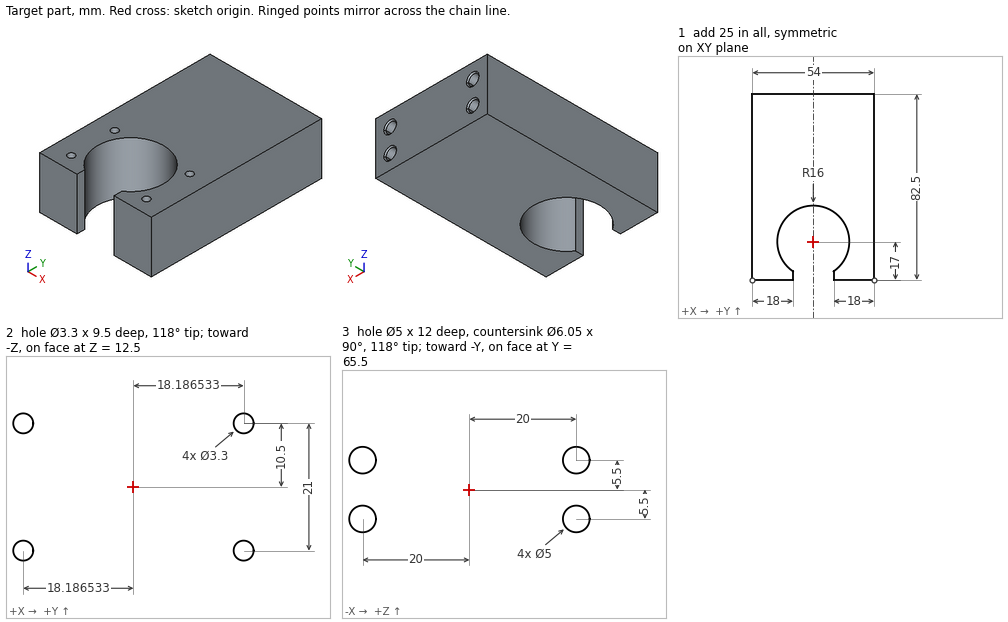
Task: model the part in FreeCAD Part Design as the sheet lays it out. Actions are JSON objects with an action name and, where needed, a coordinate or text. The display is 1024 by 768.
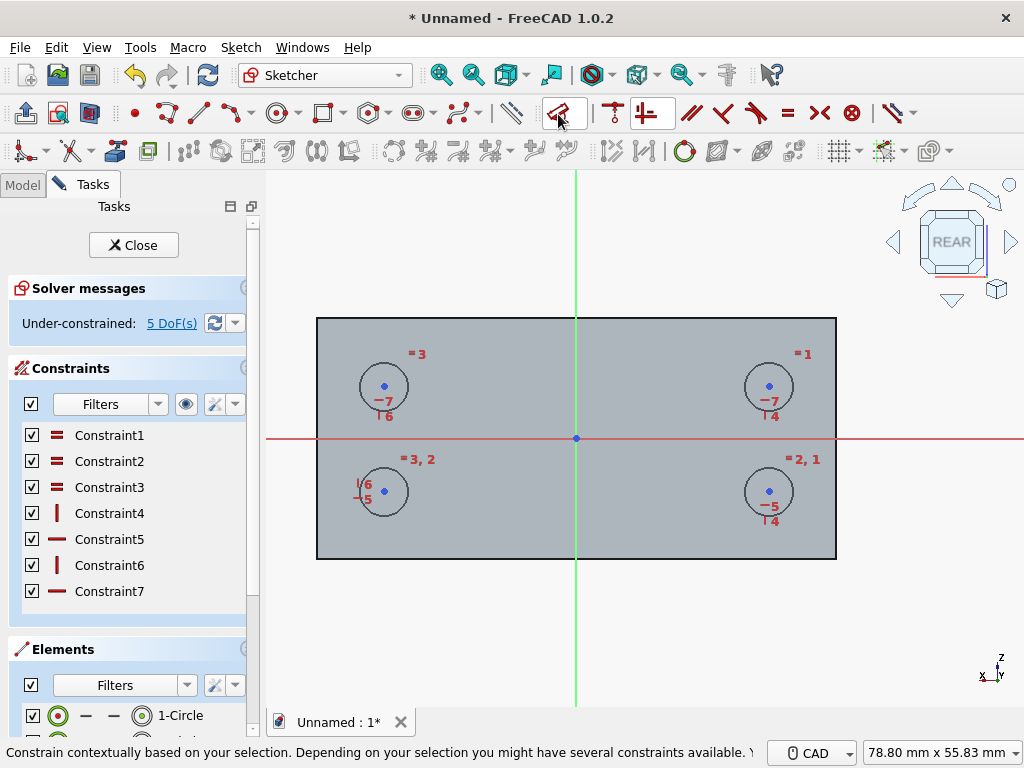
{"action": "left_click", "coordinate": [786, 370]}
{"action": "left_click", "coordinate": [809, 347]}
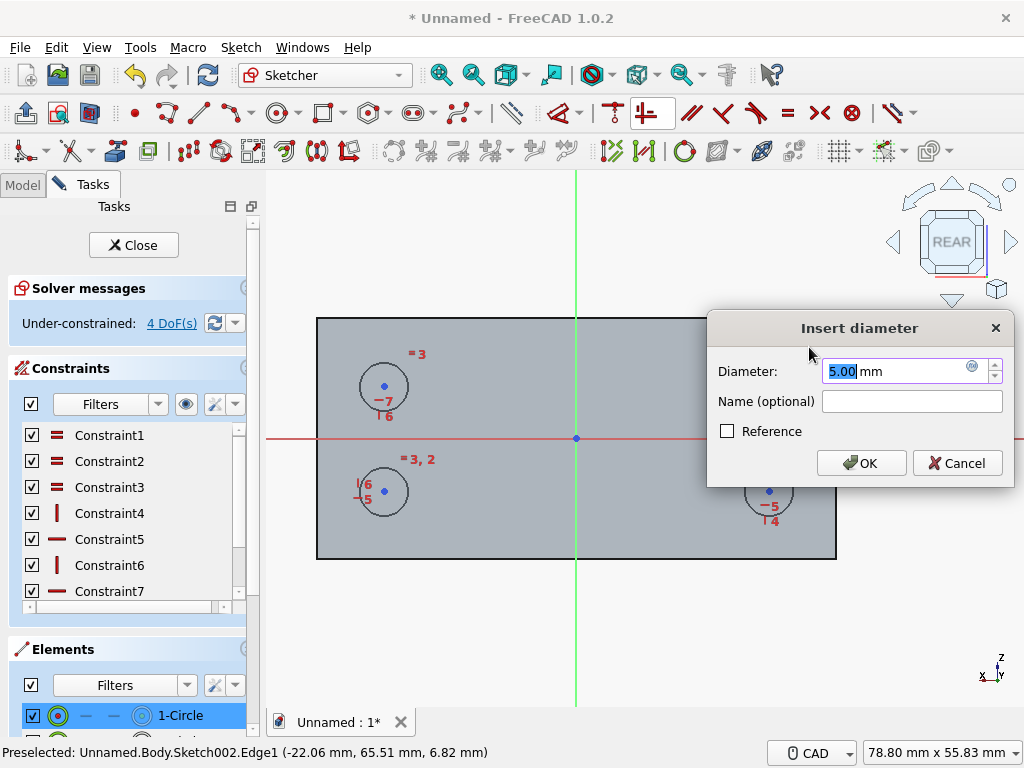
{"action": "type", "text": "5"}
{"action": "key", "text": "Return"}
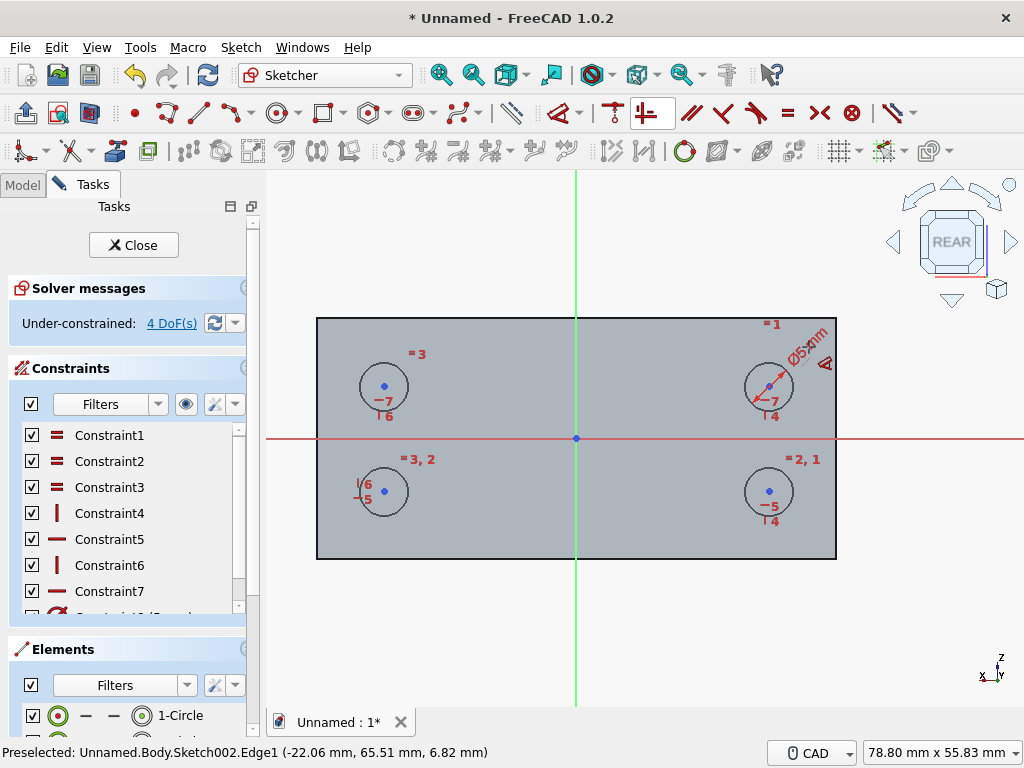
{"action": "left_click", "coordinate": [769, 387]}
{"action": "left_click", "coordinate": [673, 353]}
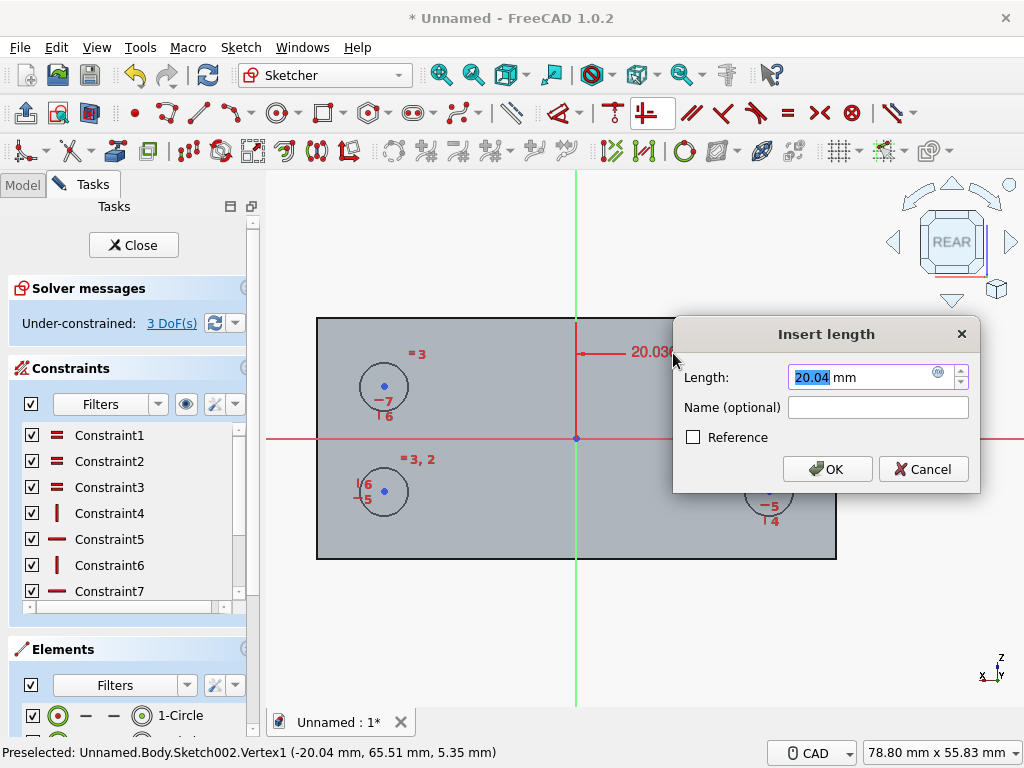
{"action": "type", "text": "20"}
{"action": "key", "text": "Return"}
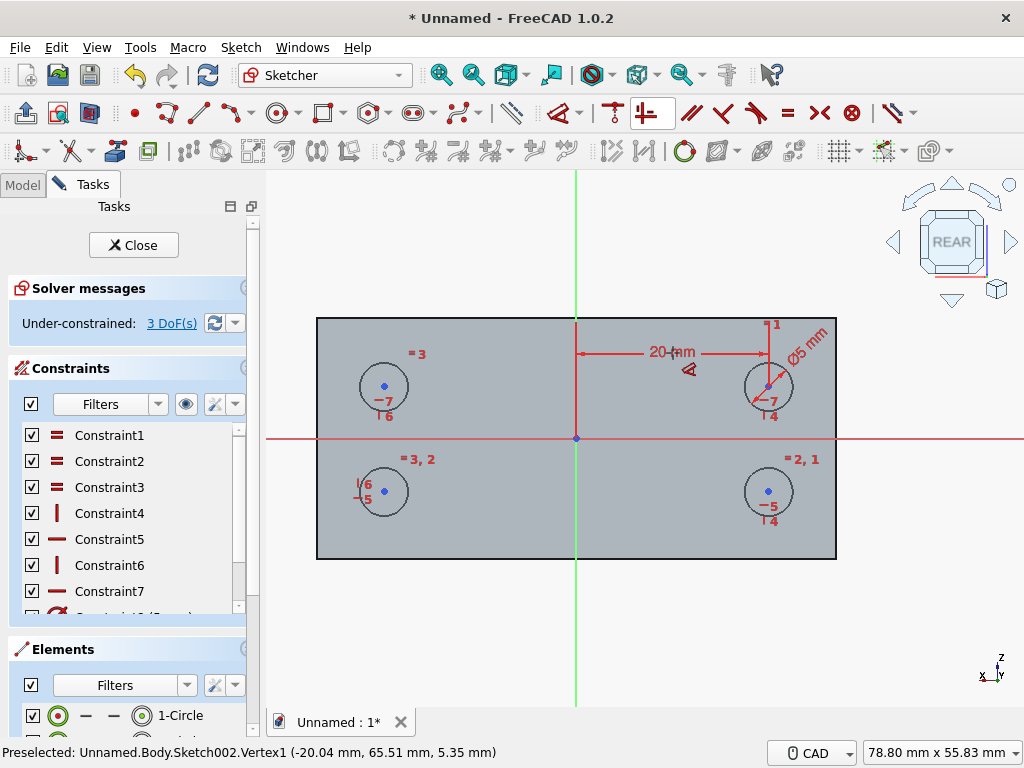
{"action": "left_click", "coordinate": [384, 492]}
{"action": "left_click", "coordinate": [480, 526]}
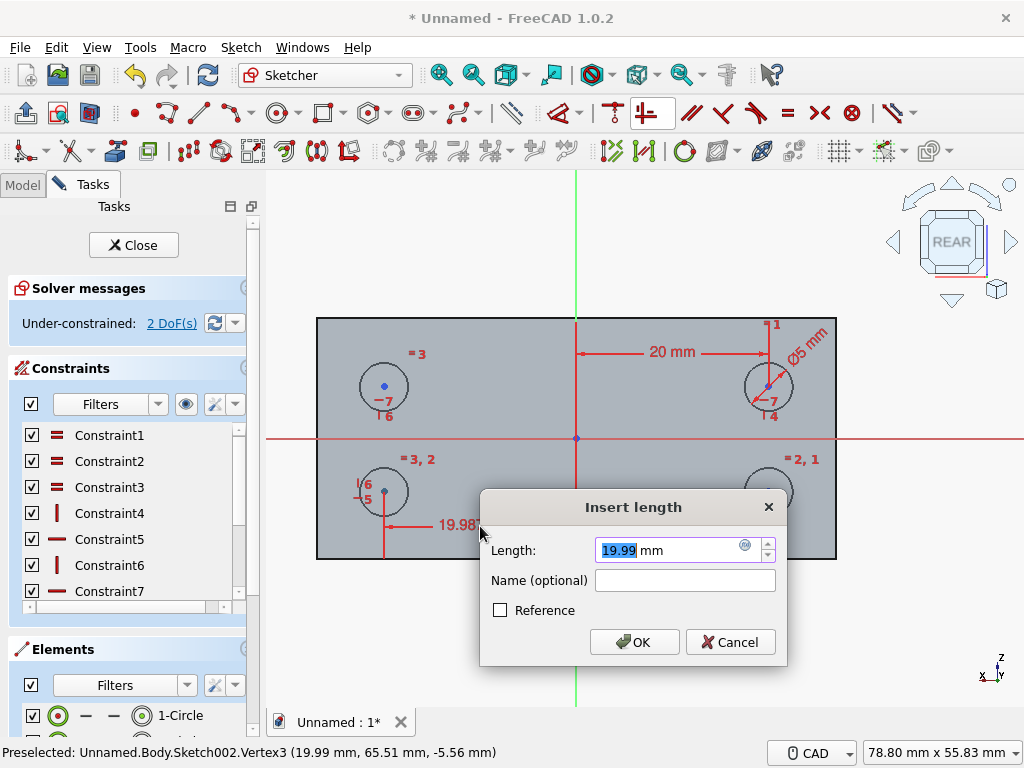
{"action": "type", "text": "20"}
{"action": "key", "text": "Return"}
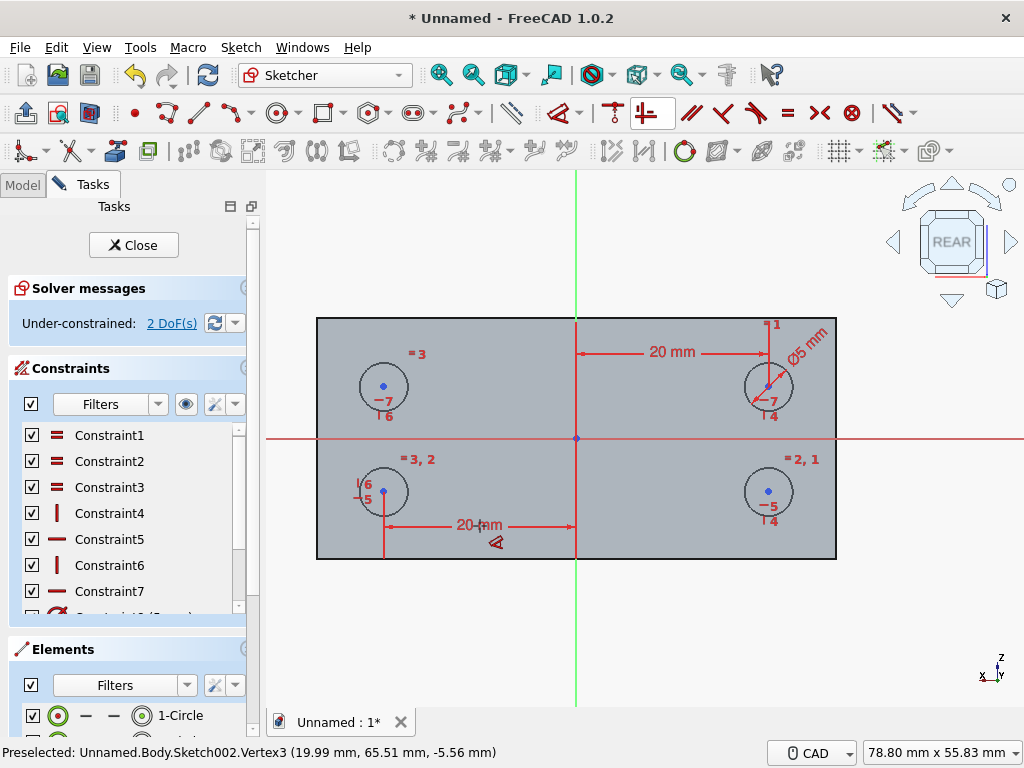
{"action": "left_click", "coordinate": [769, 387]}
{"action": "left_click", "coordinate": [803, 413]}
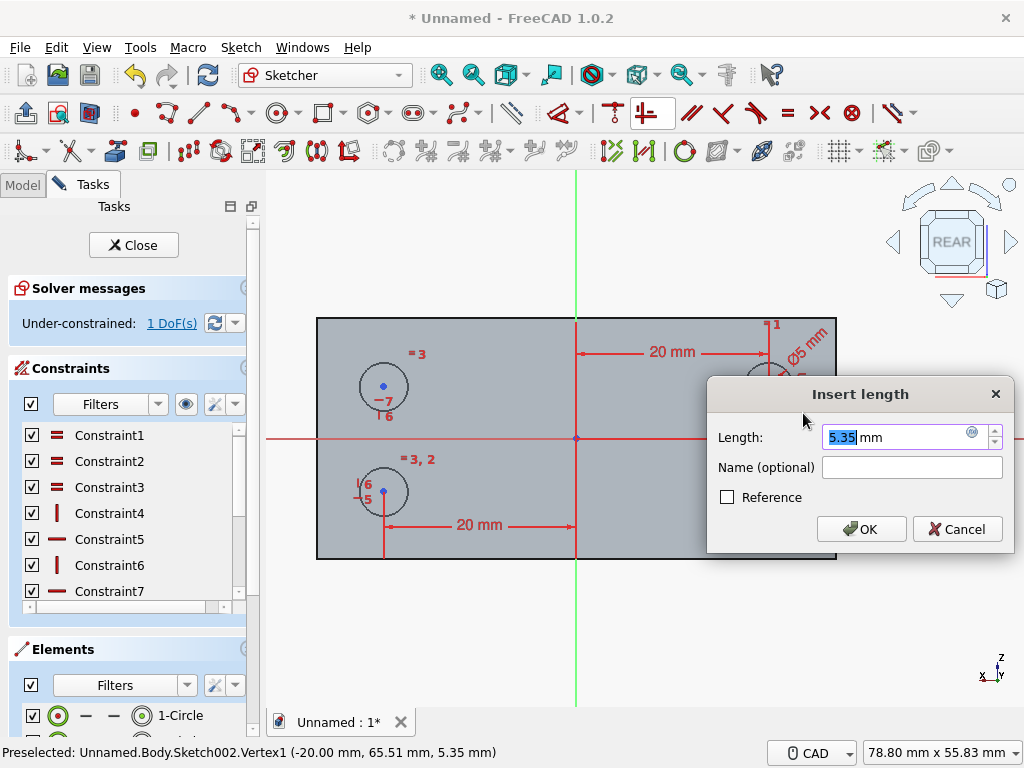
{"action": "type", "text": "5.5"}
{"action": "key", "text": "Return"}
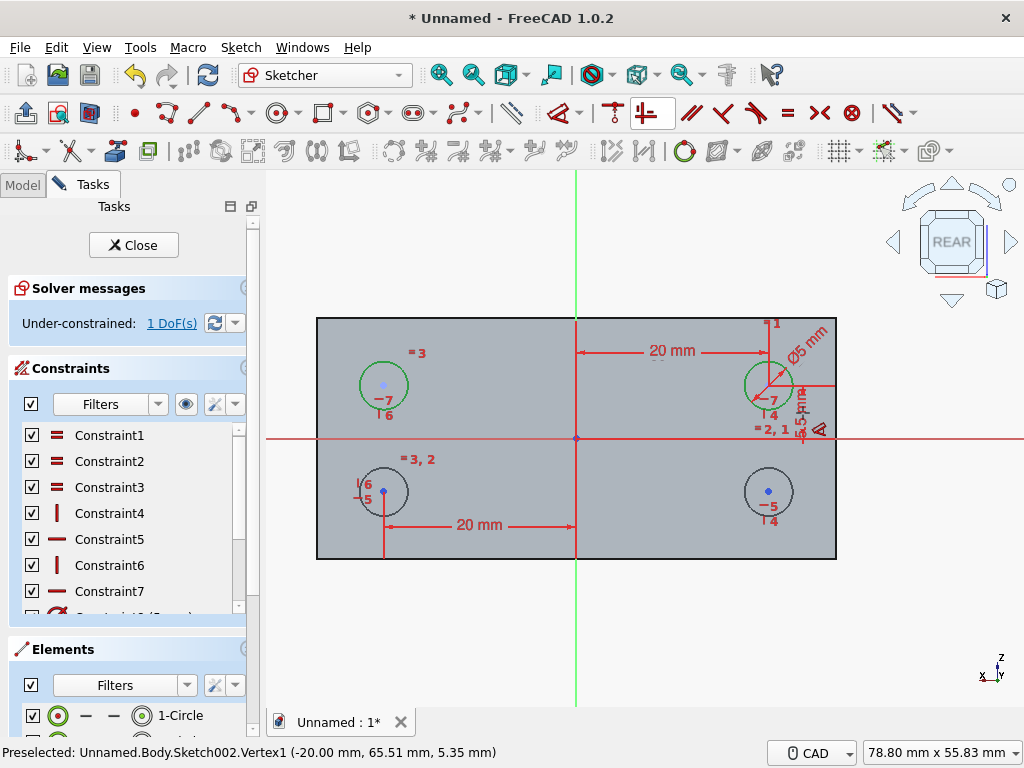
{"action": "left_click", "coordinate": [769, 492]}
{"action": "left_click", "coordinate": [803, 465]}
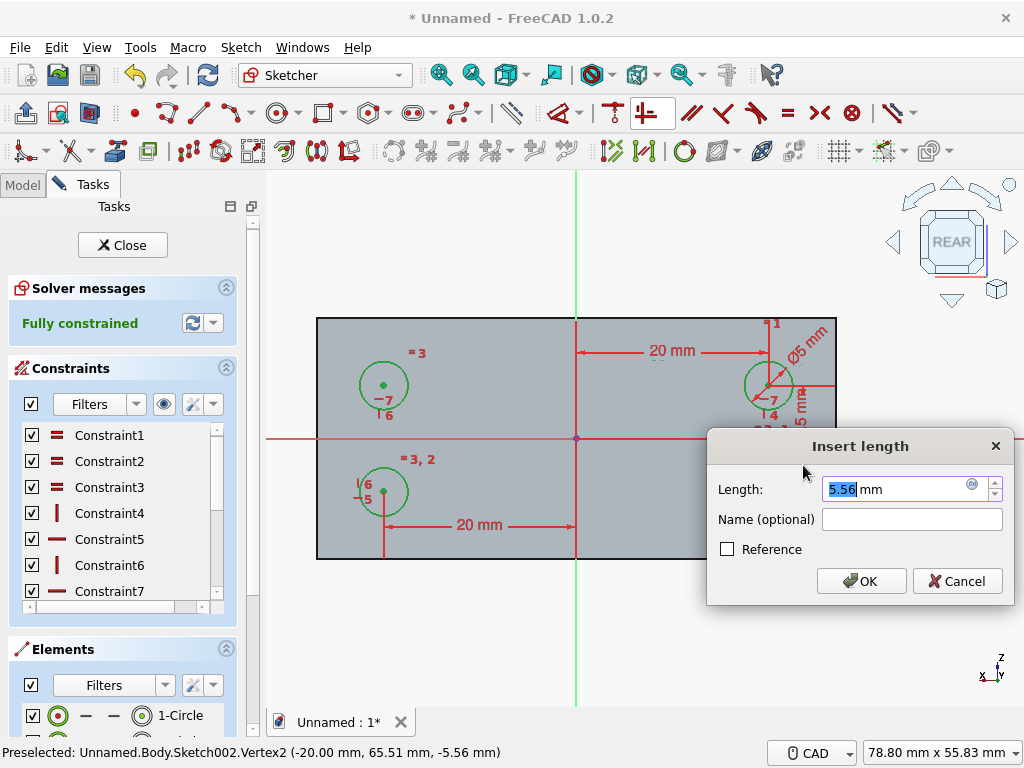
{"action": "type", "text": "5.5"}
{"action": "key", "text": "Return"}
{"action": "key", "text": "Escape"}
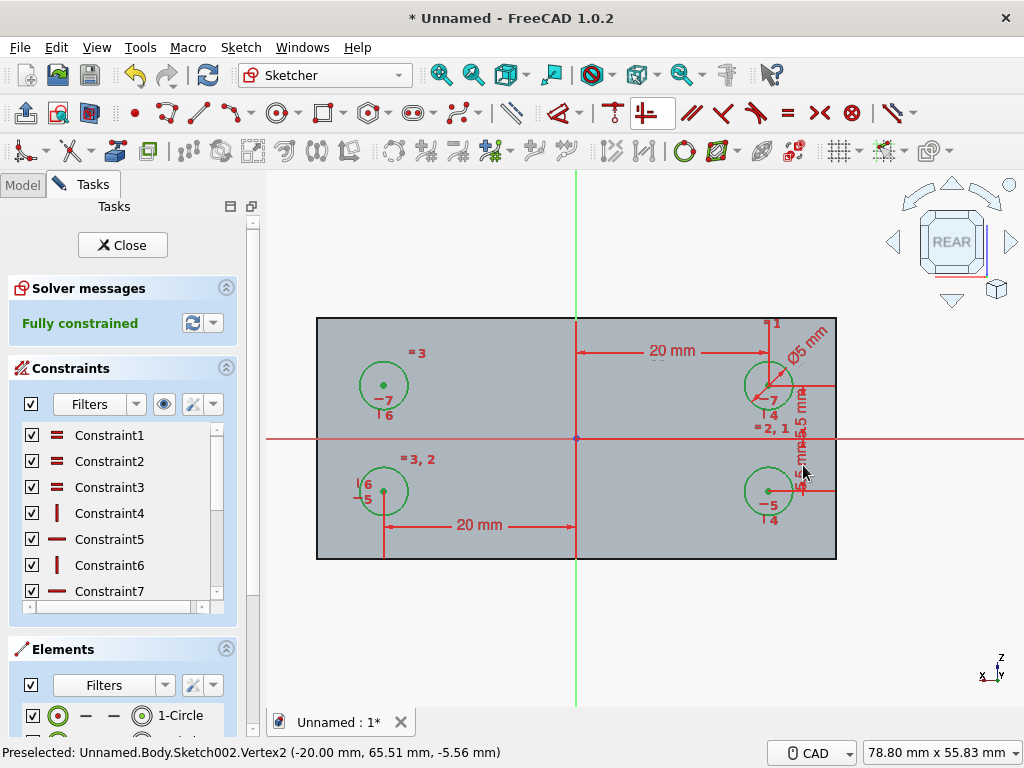
{"action": "left_click", "coordinate": [123, 245]}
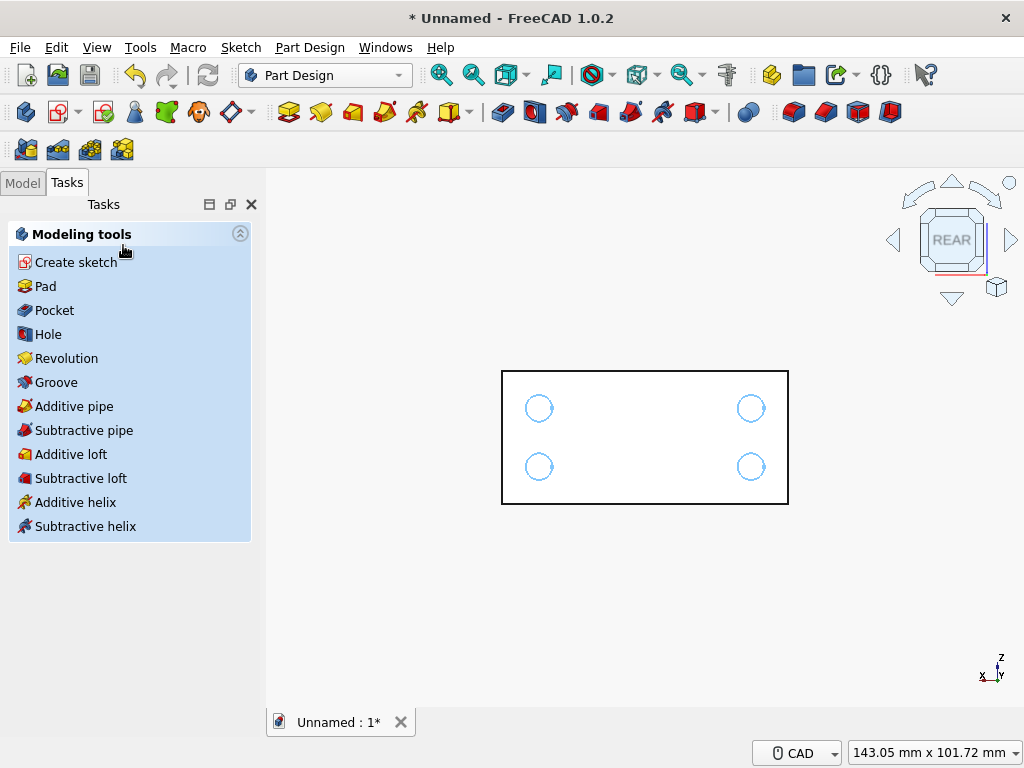
{"action": "left_click", "coordinate": [536, 112]}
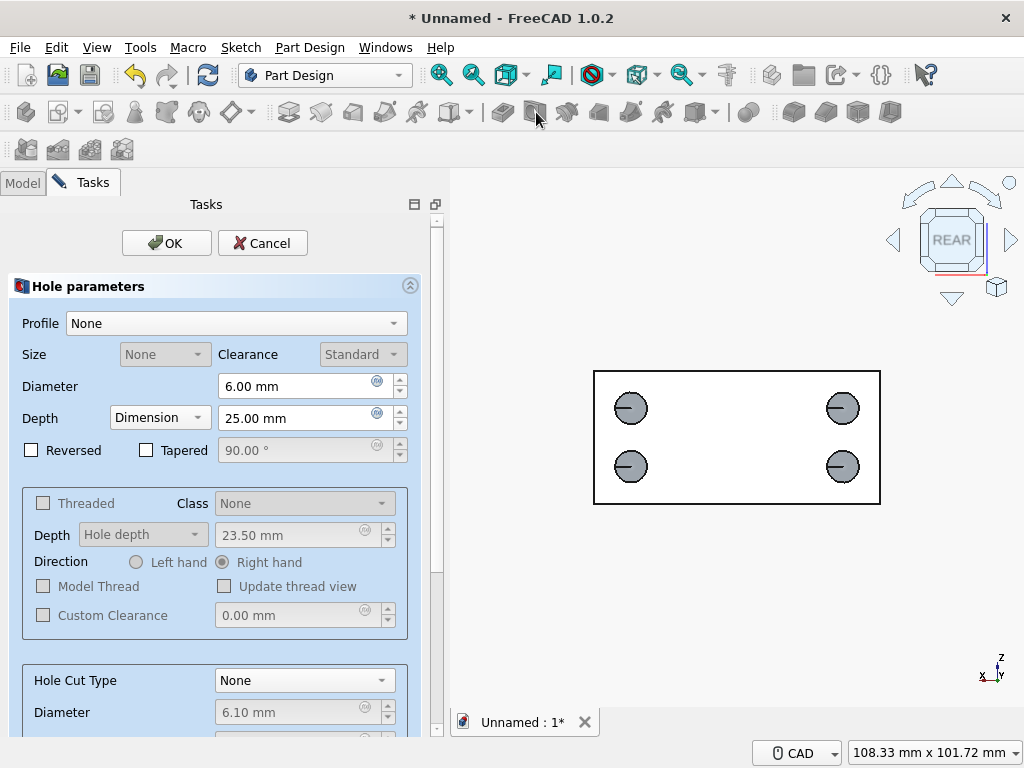
{"action": "triple_click", "coordinate": [305, 386]}